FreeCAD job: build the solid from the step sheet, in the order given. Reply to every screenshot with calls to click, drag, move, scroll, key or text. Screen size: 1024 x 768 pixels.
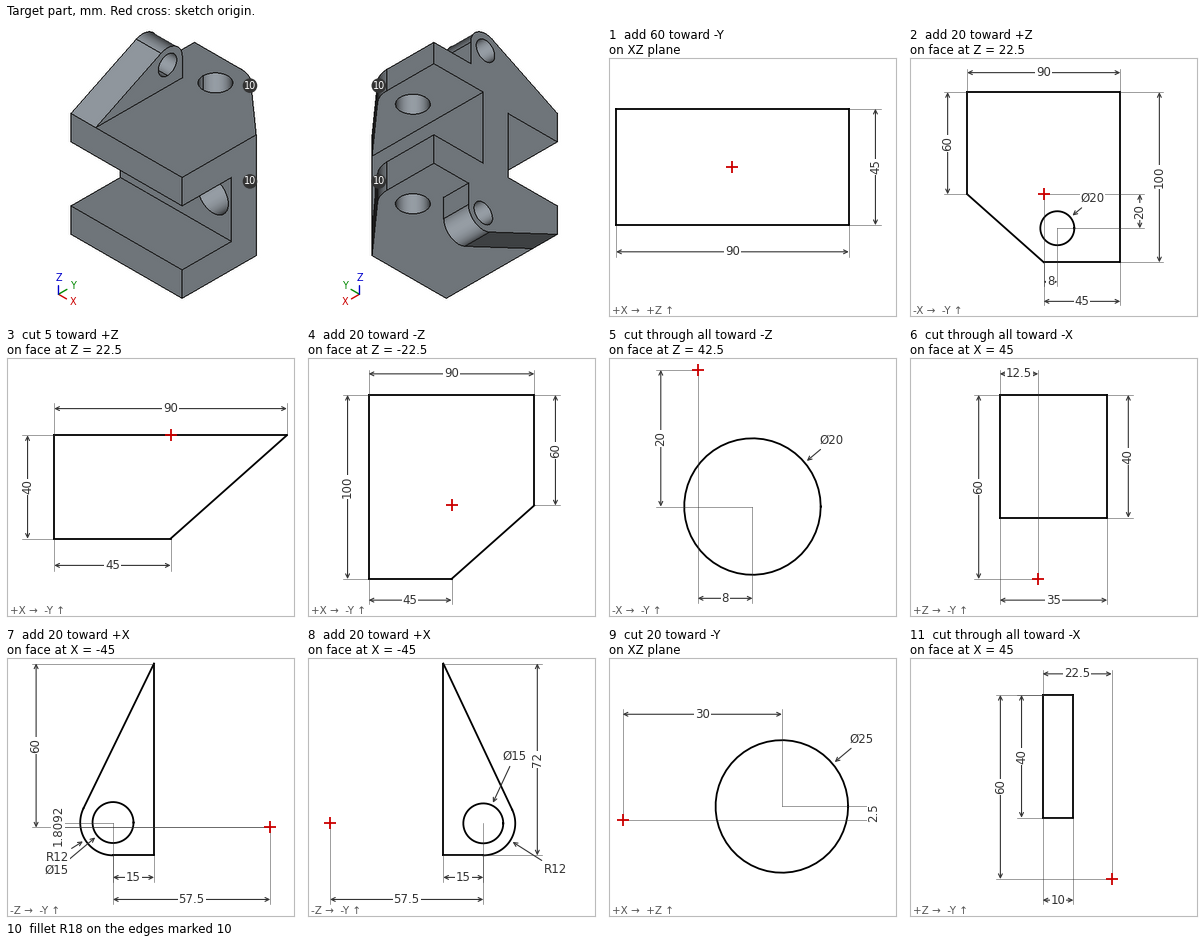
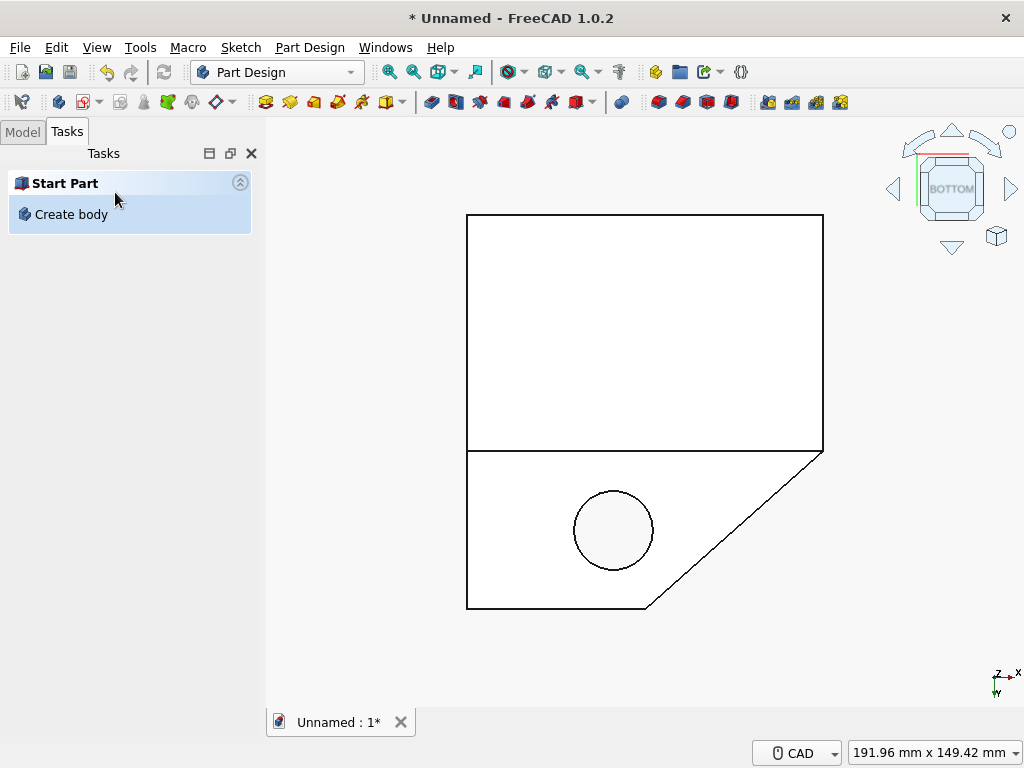
click(696, 332)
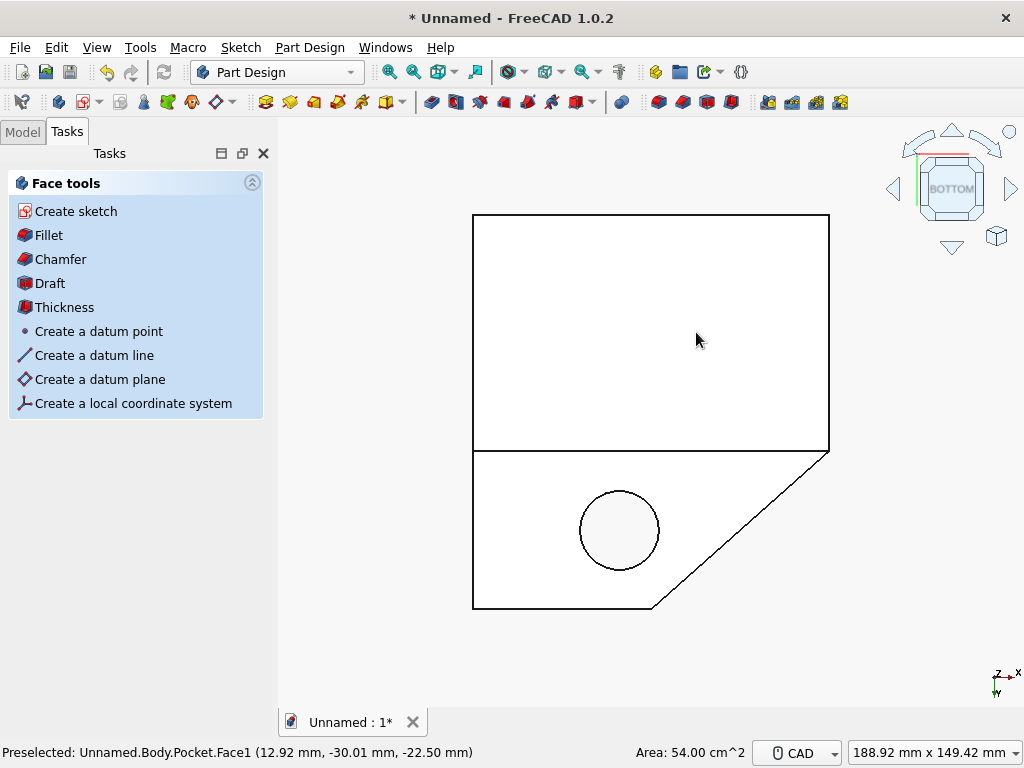
click(84, 102)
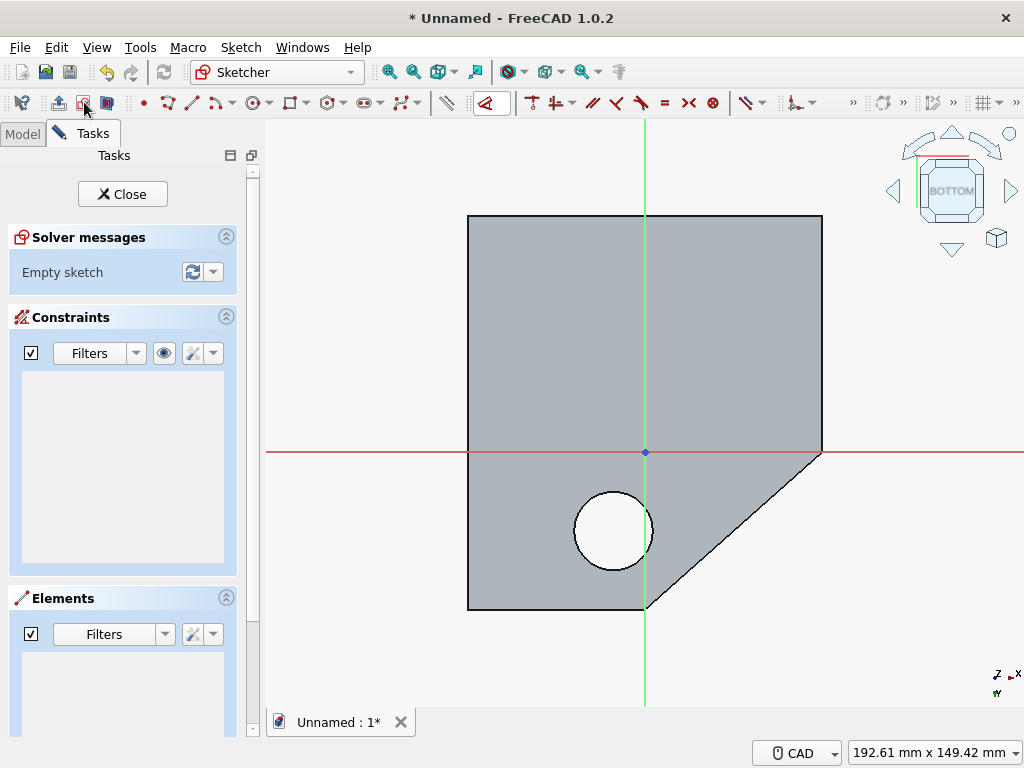
key(g)
key(m)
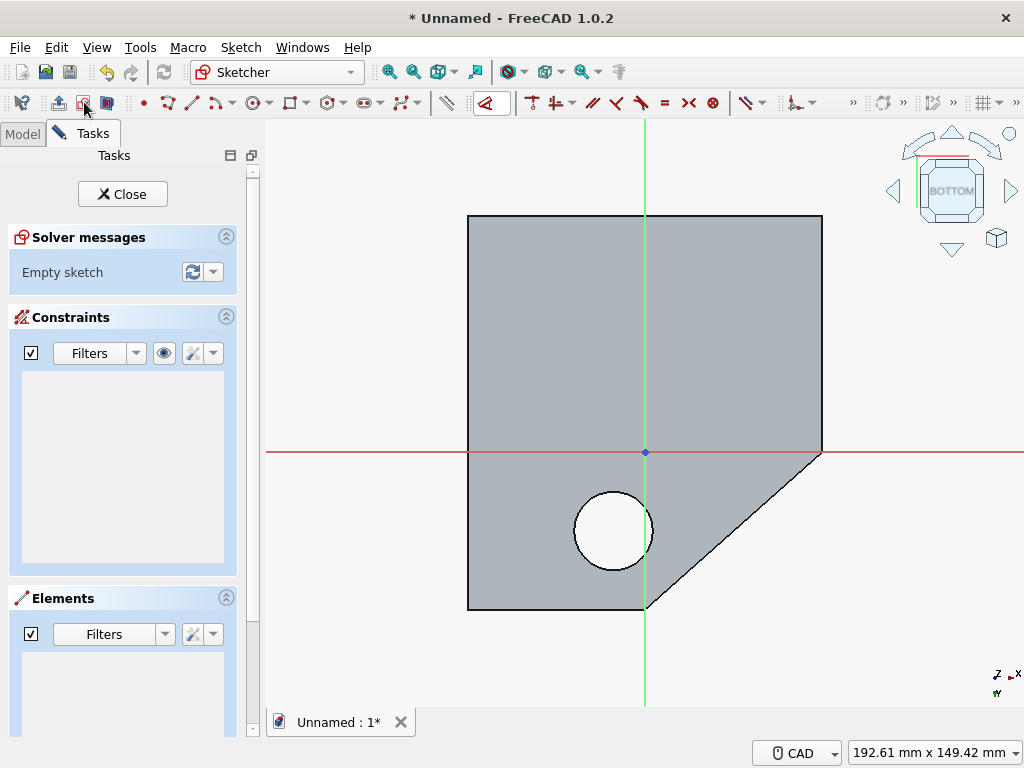
click(645, 610)
click(822, 452)
click(822, 216)
click(468, 216)
click(468, 610)
click(645, 611)
key(Escape)
key(Escape)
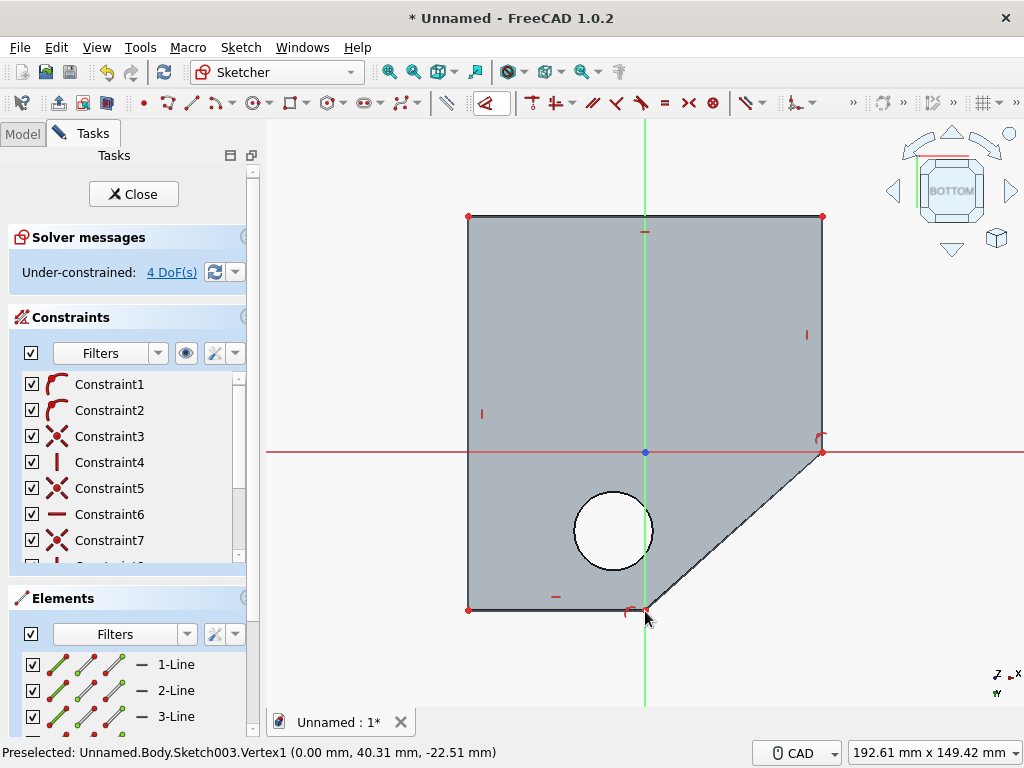
click(822, 382)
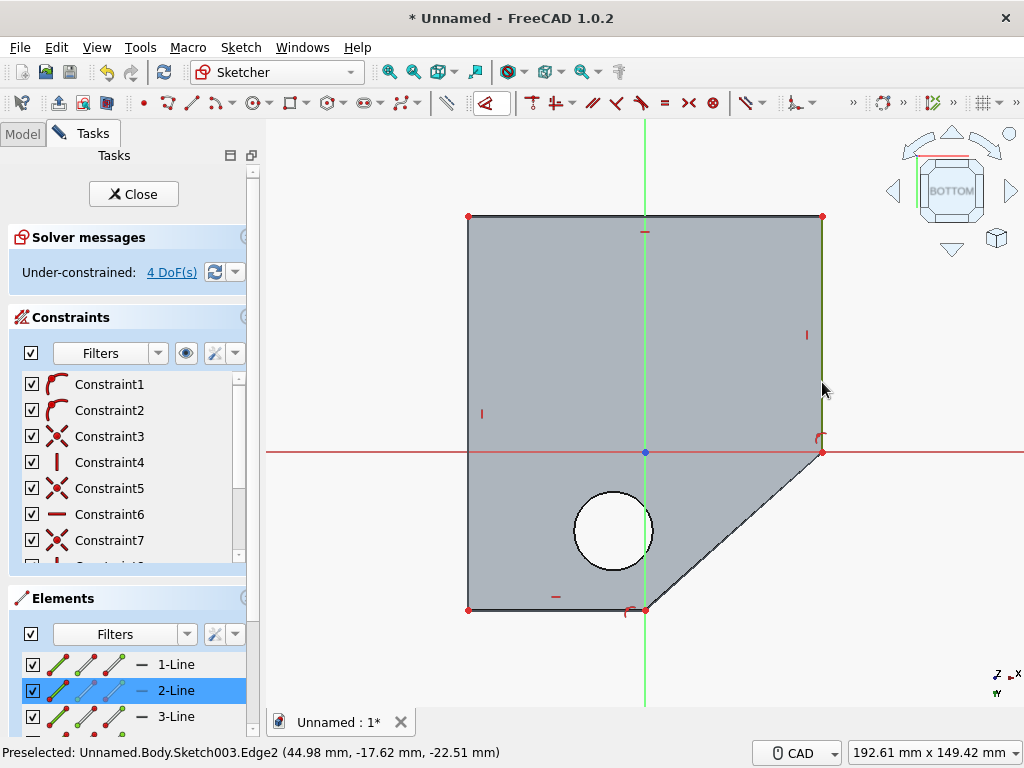
key(i)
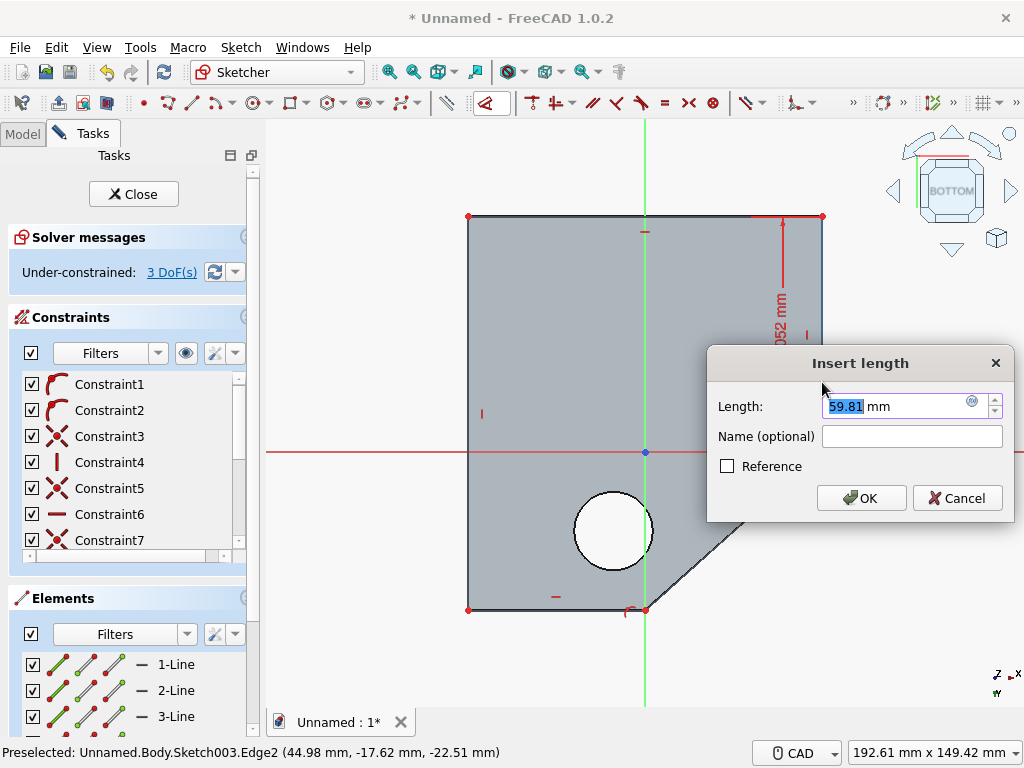
text(60)
key(Return)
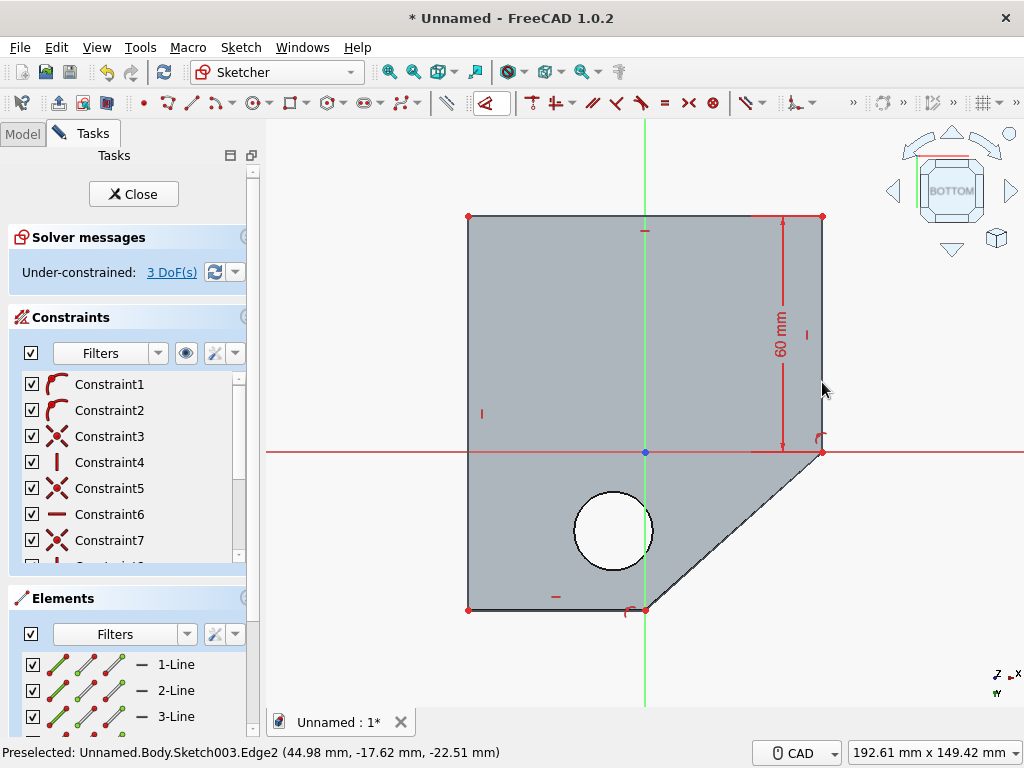
click(716, 216)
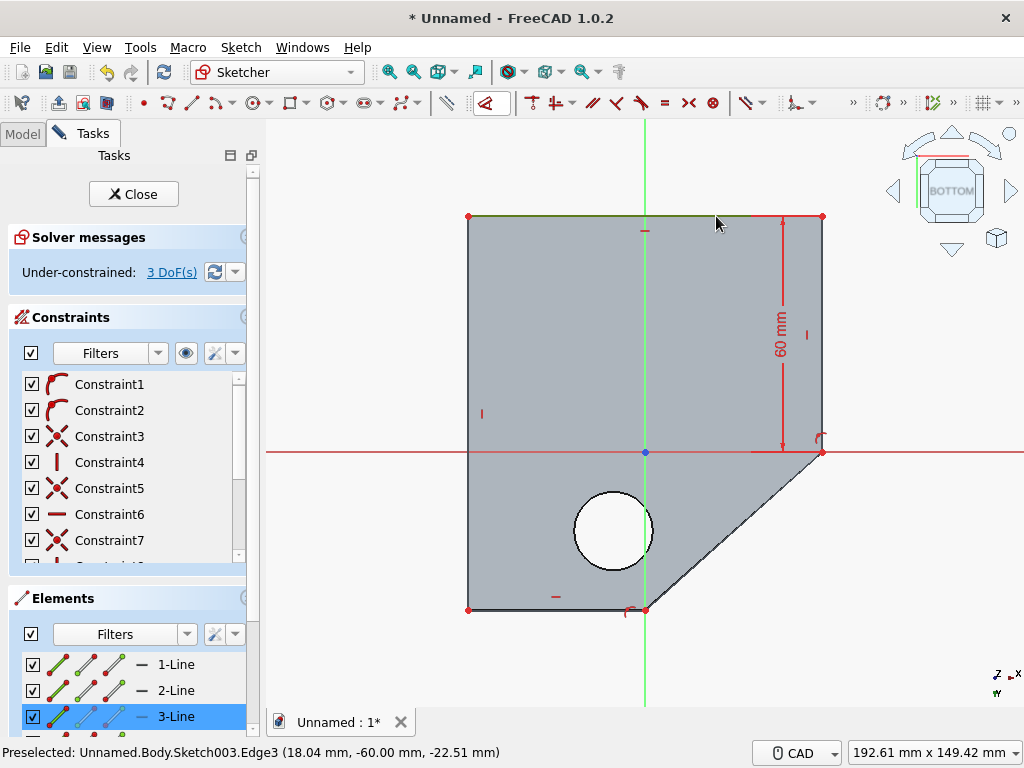
key(l)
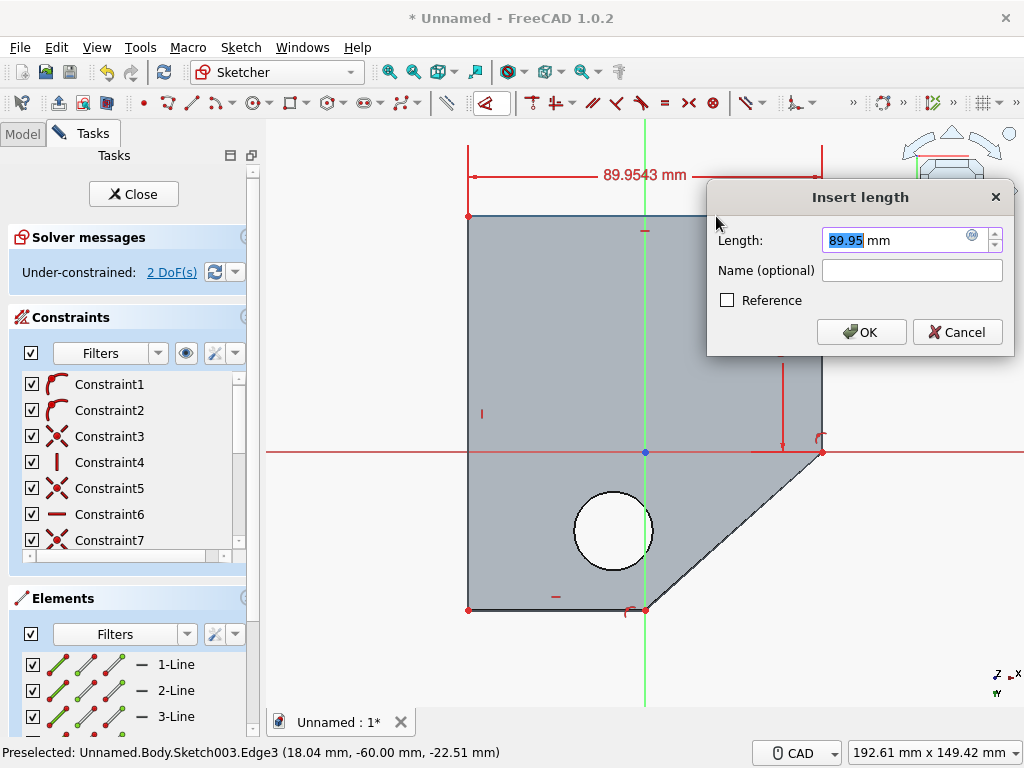
text(90)
key(Return)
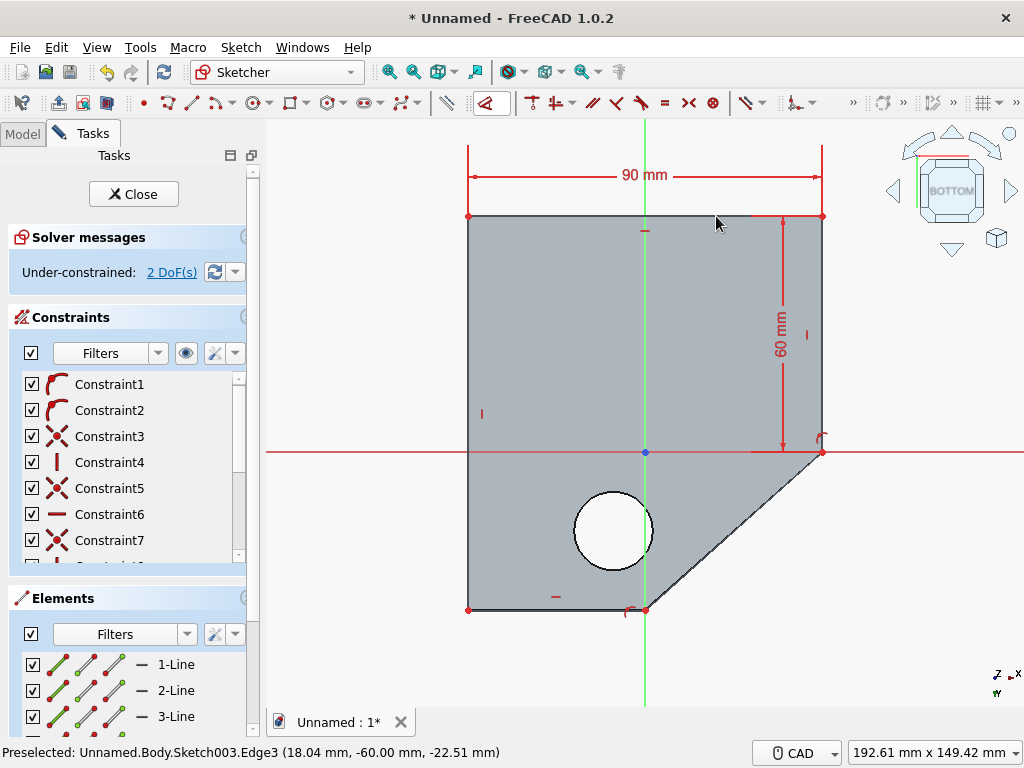
click(521, 611)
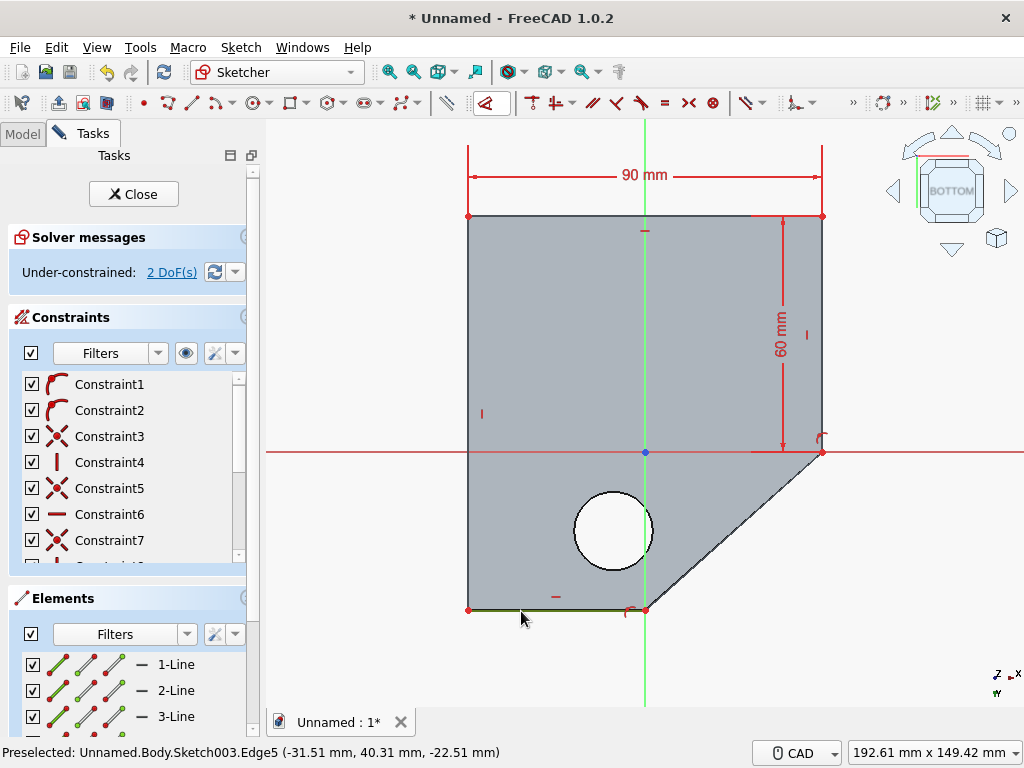
key(l)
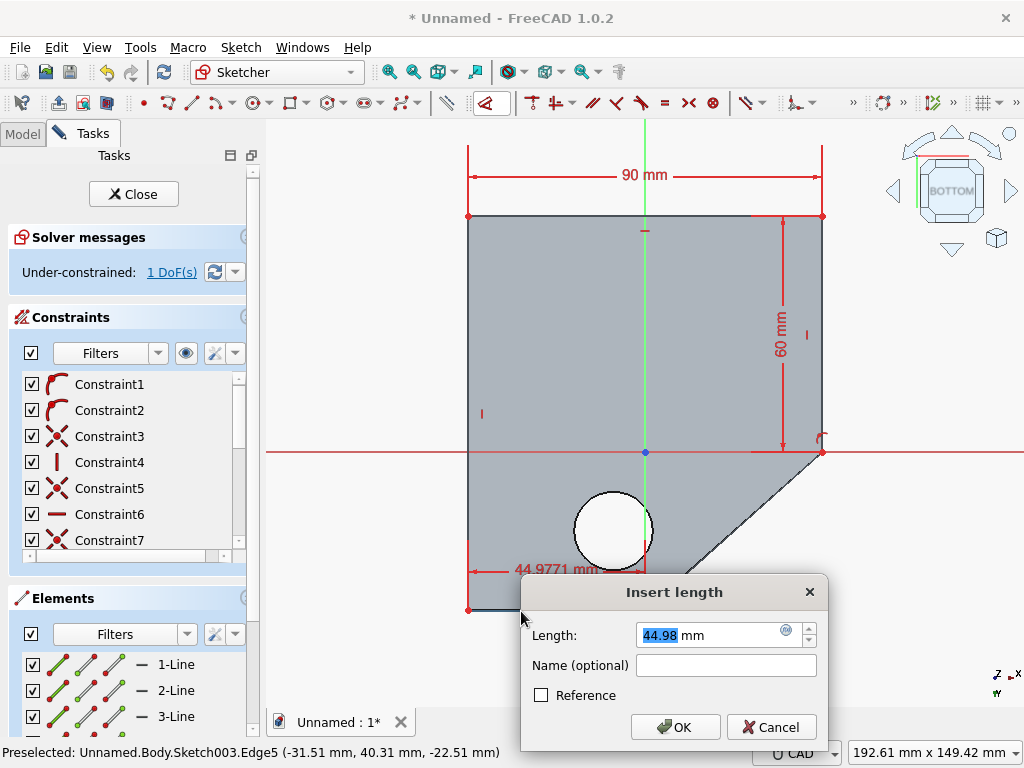
text(45)
key(Return)